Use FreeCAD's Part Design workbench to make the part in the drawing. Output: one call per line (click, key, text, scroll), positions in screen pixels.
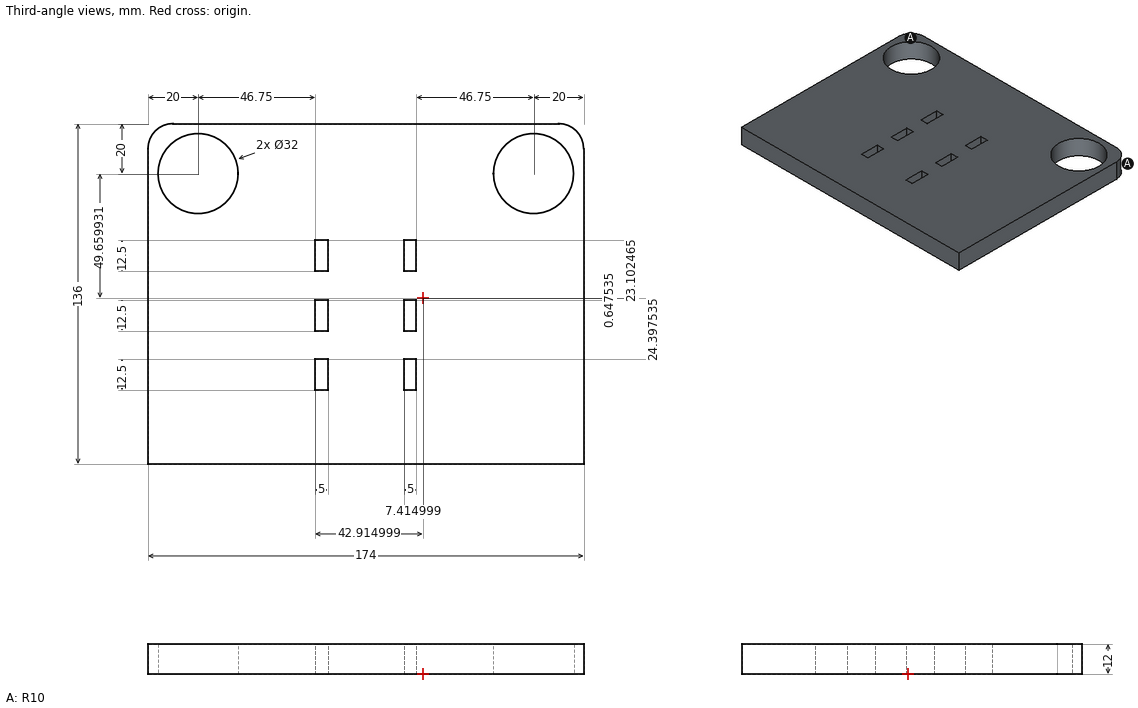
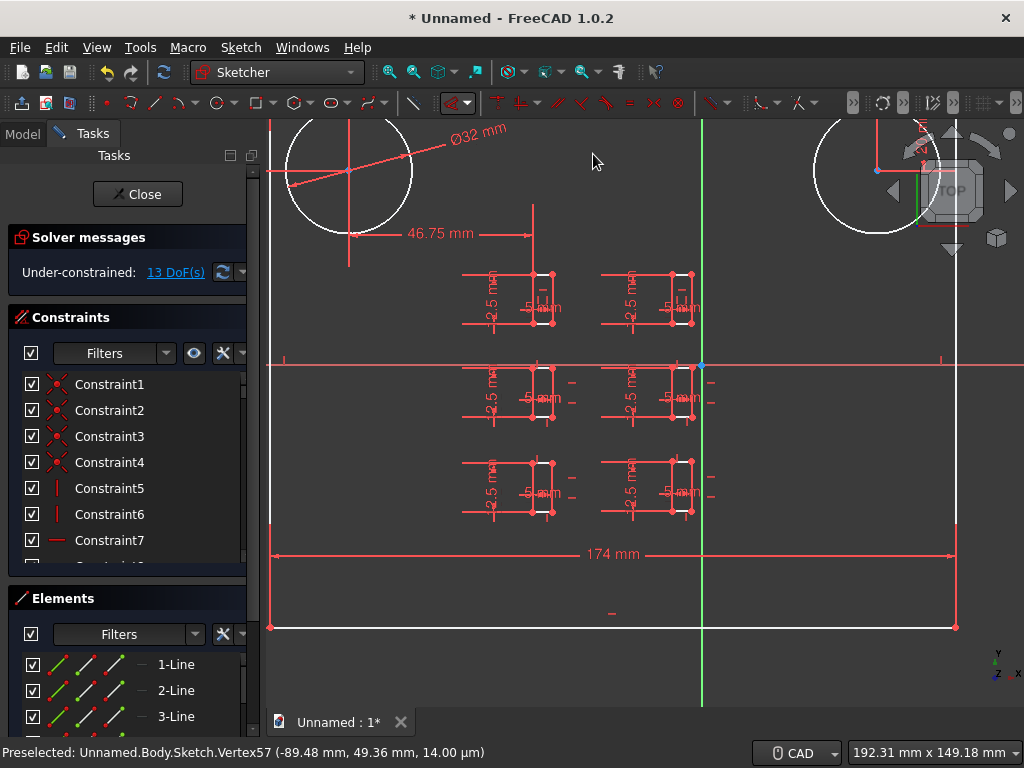
click(692, 275)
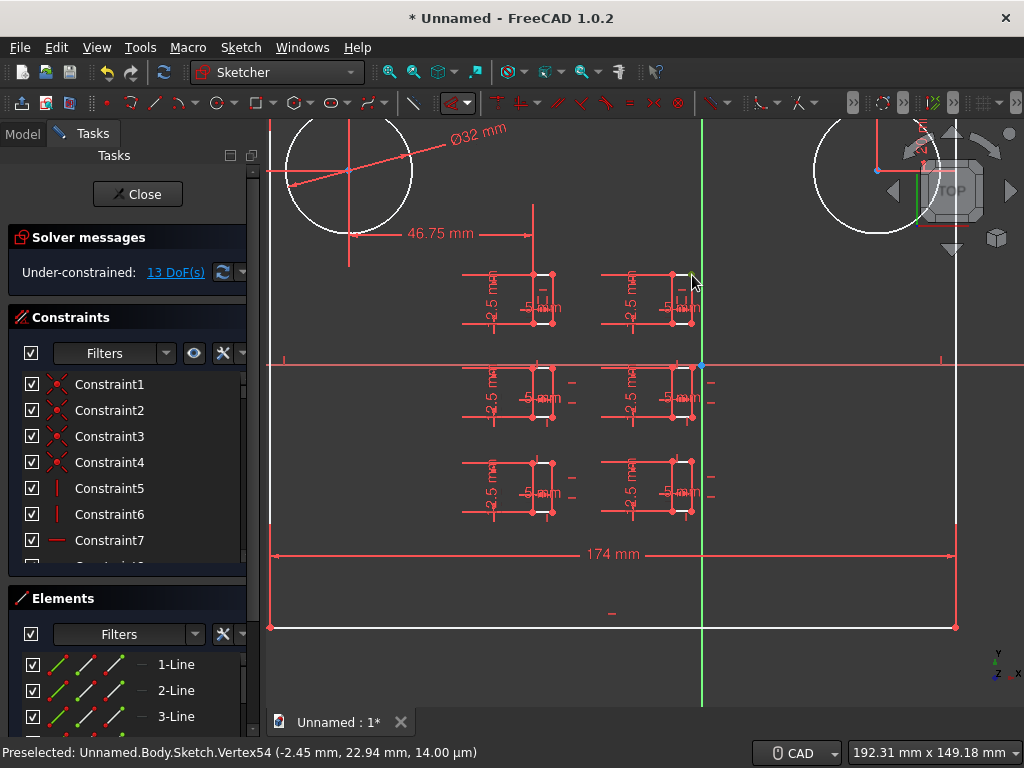
scroll(533, 479, down, 3)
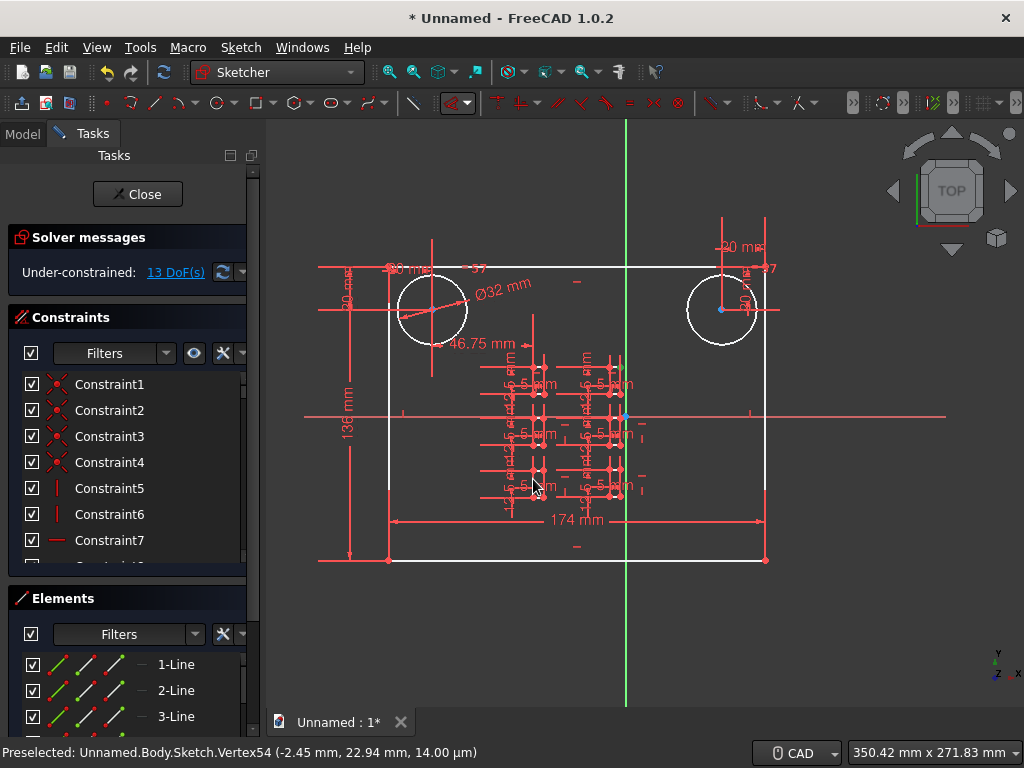
click(722, 310)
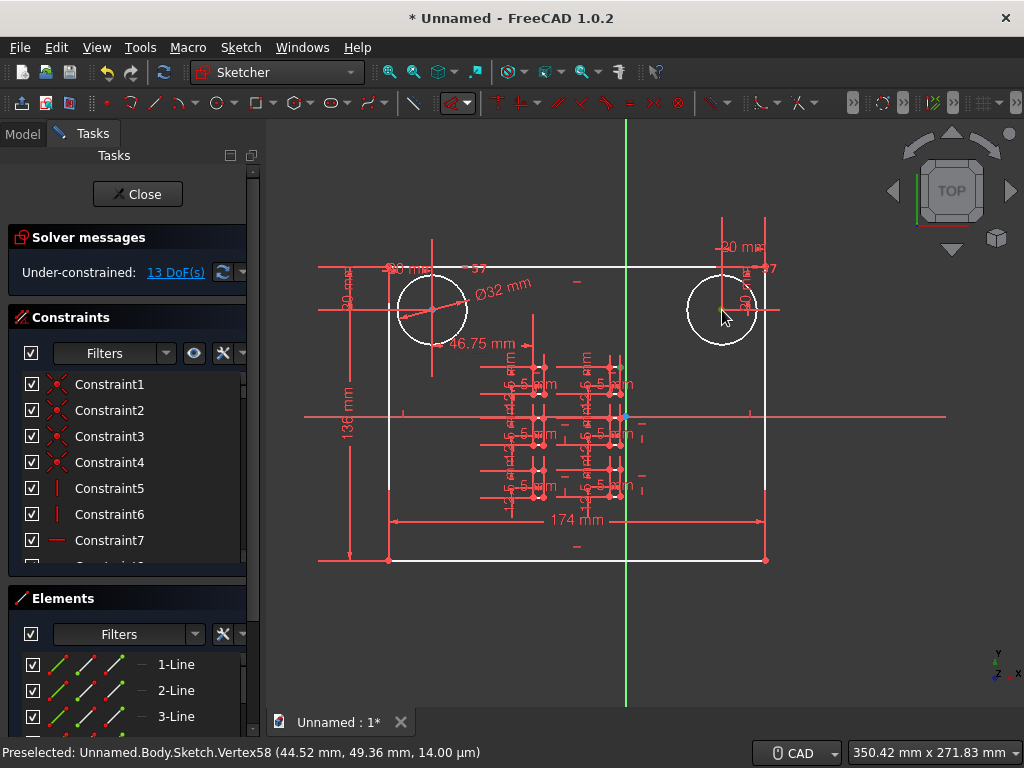
key(l)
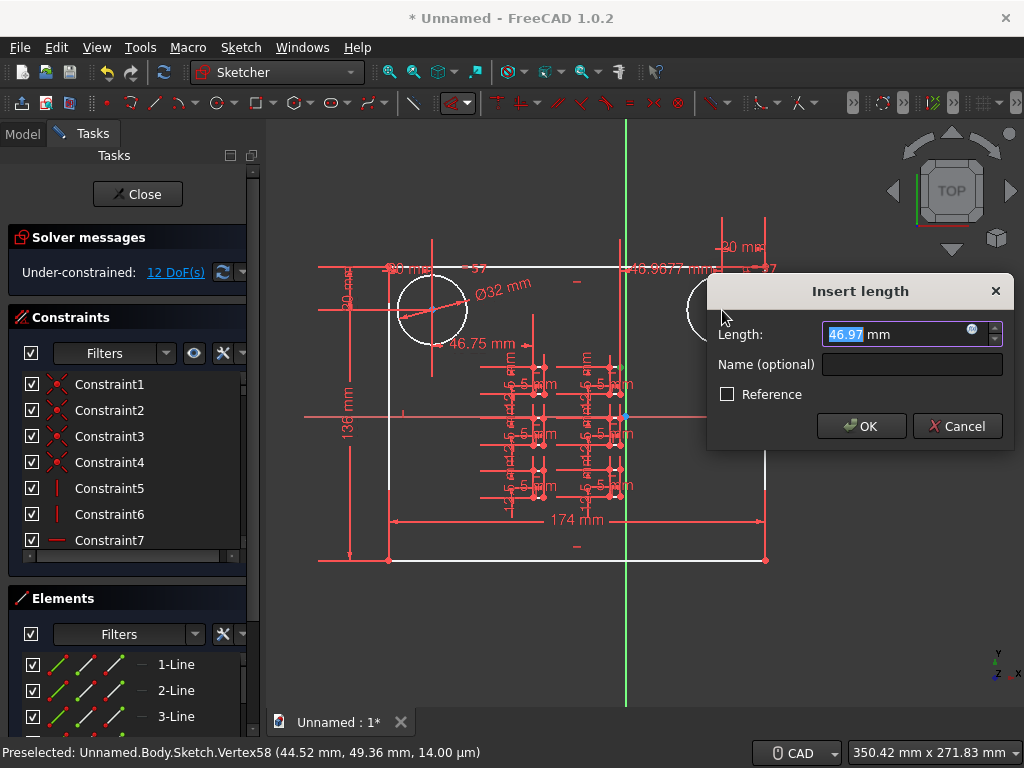
text(46.75)
key(Return)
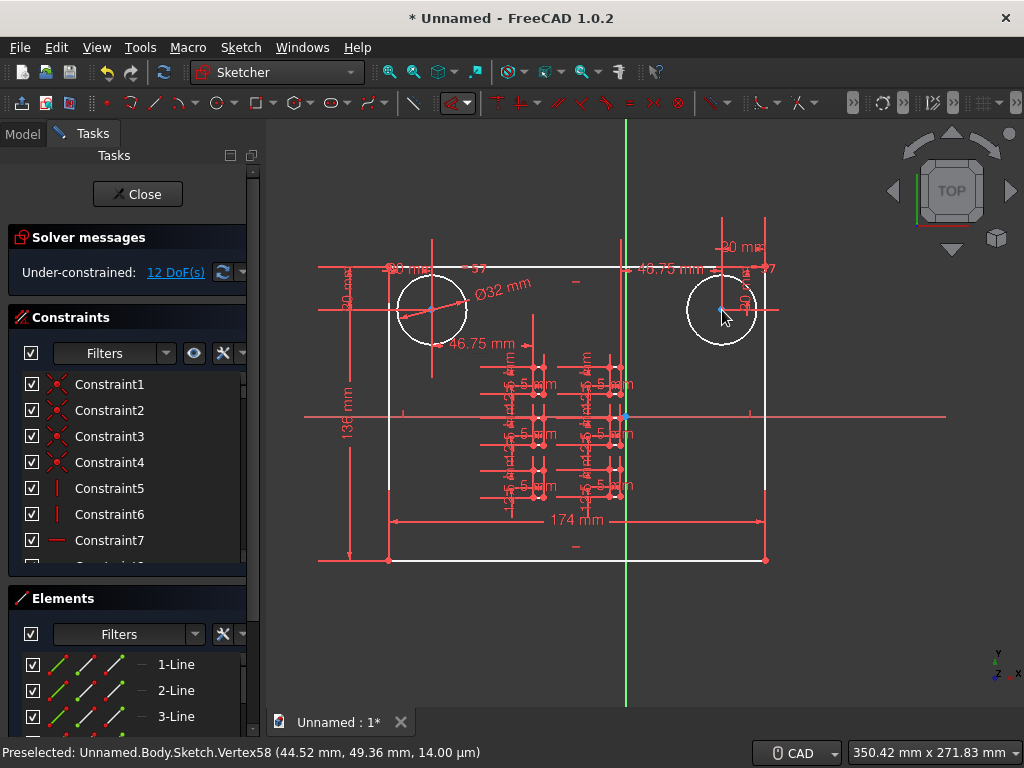
scroll(533, 418, up, 17)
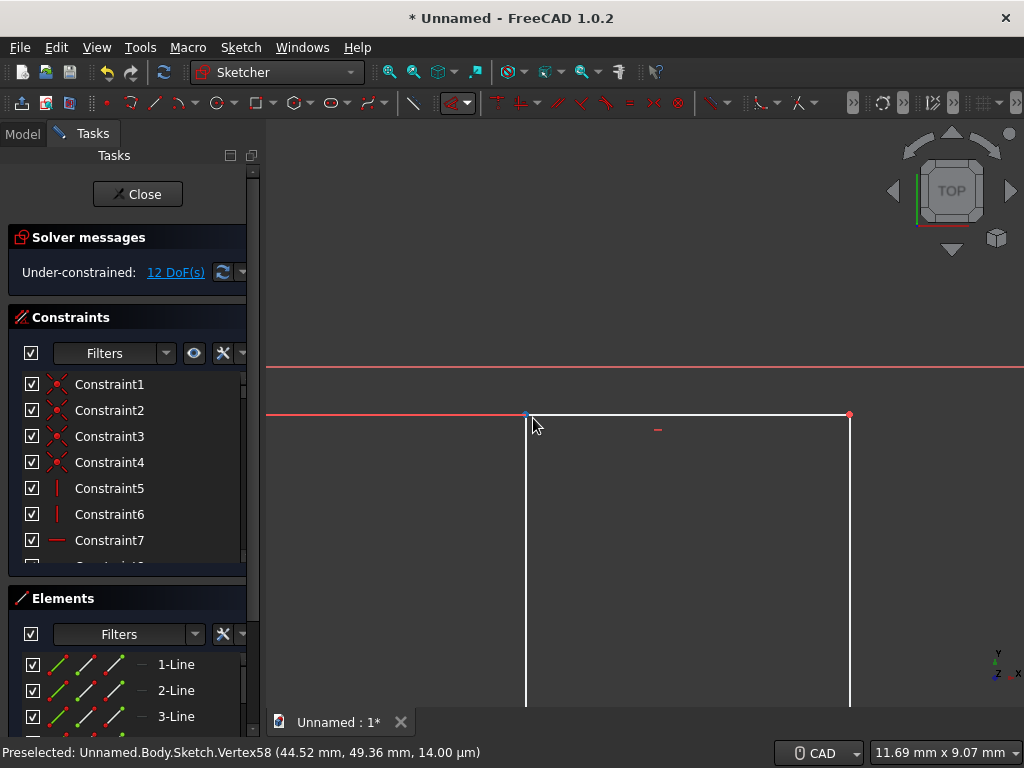
click(526, 415)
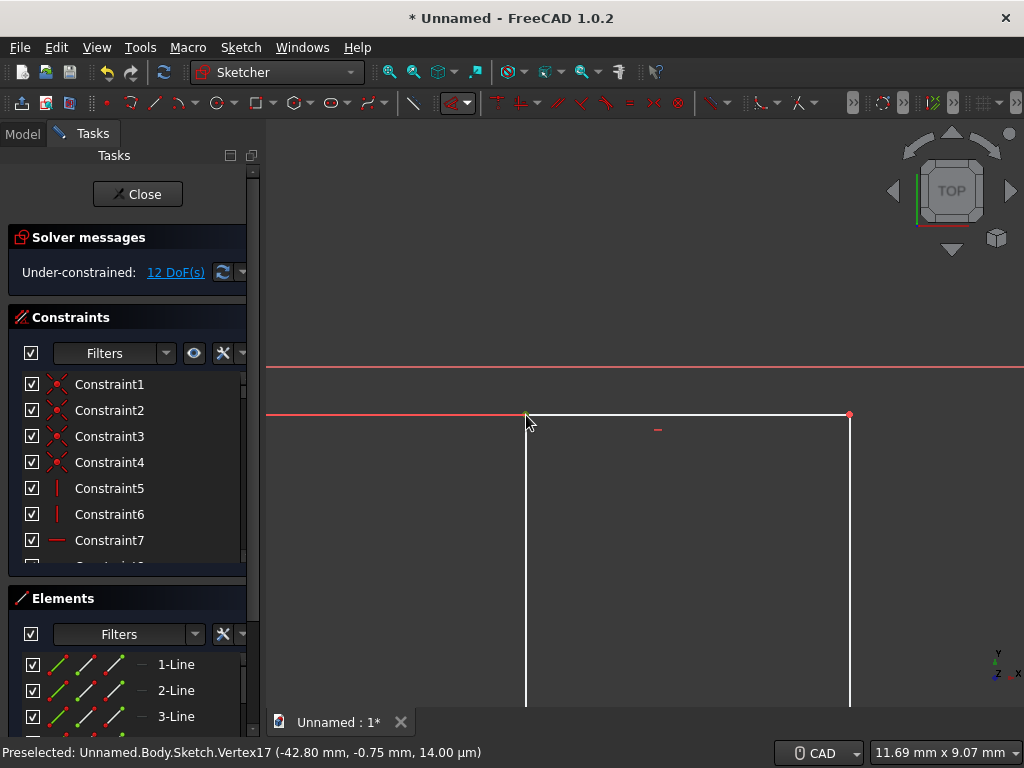
click(470, 104)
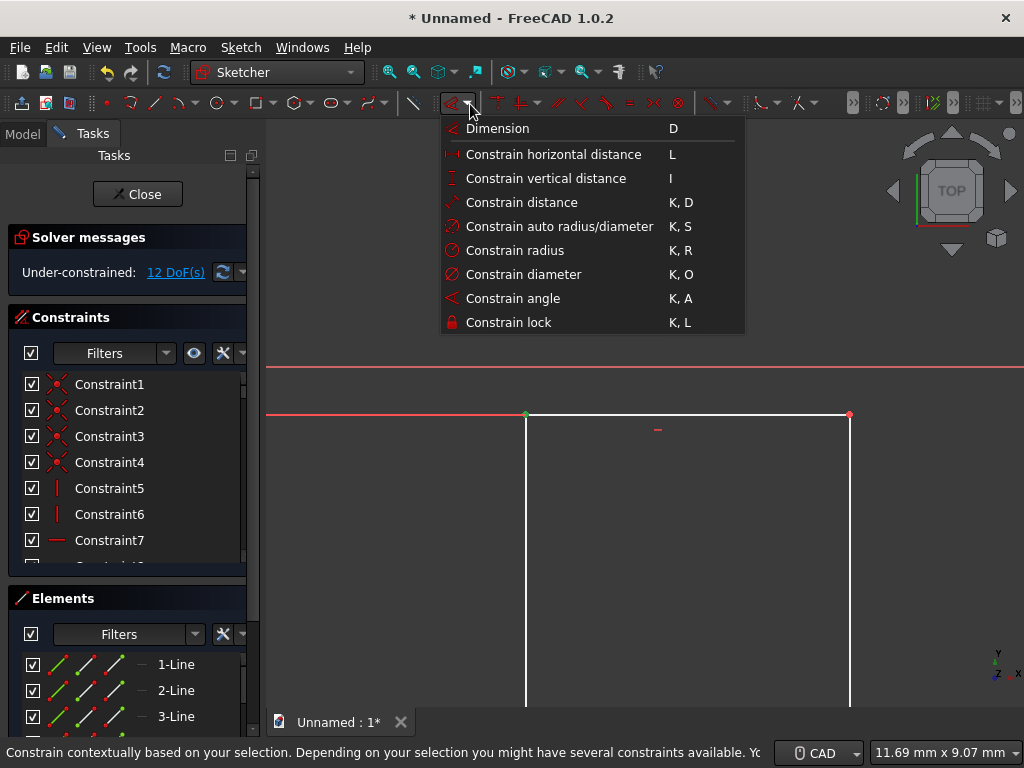
click(593, 178)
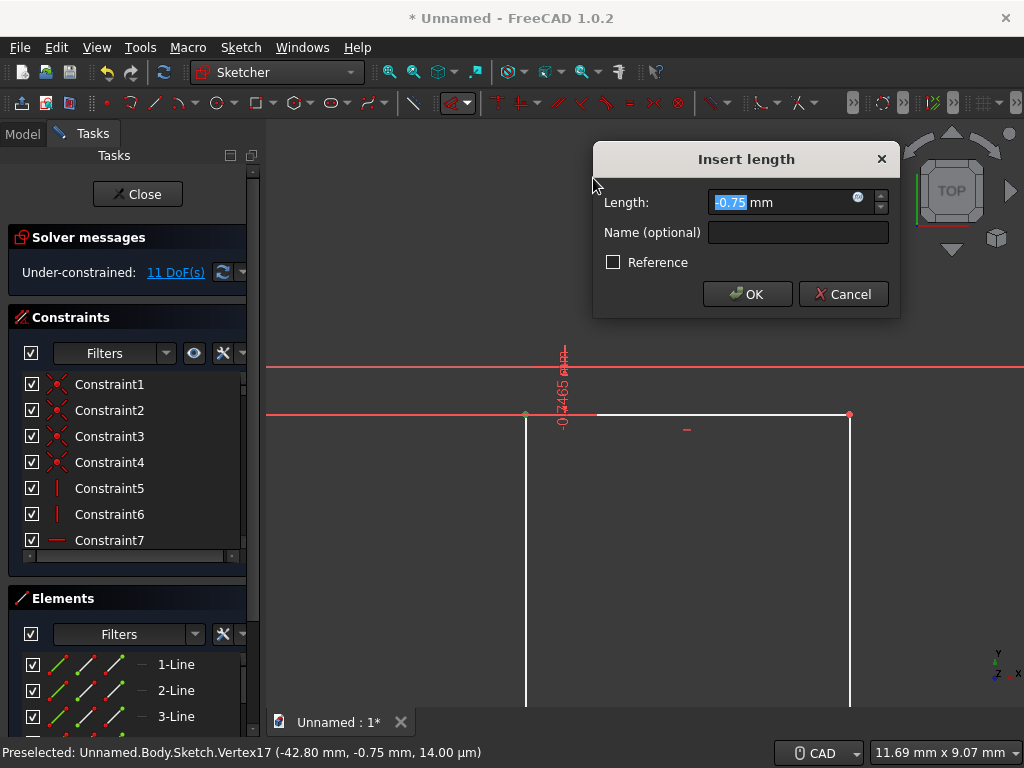
text(-0.647535)
key(Return)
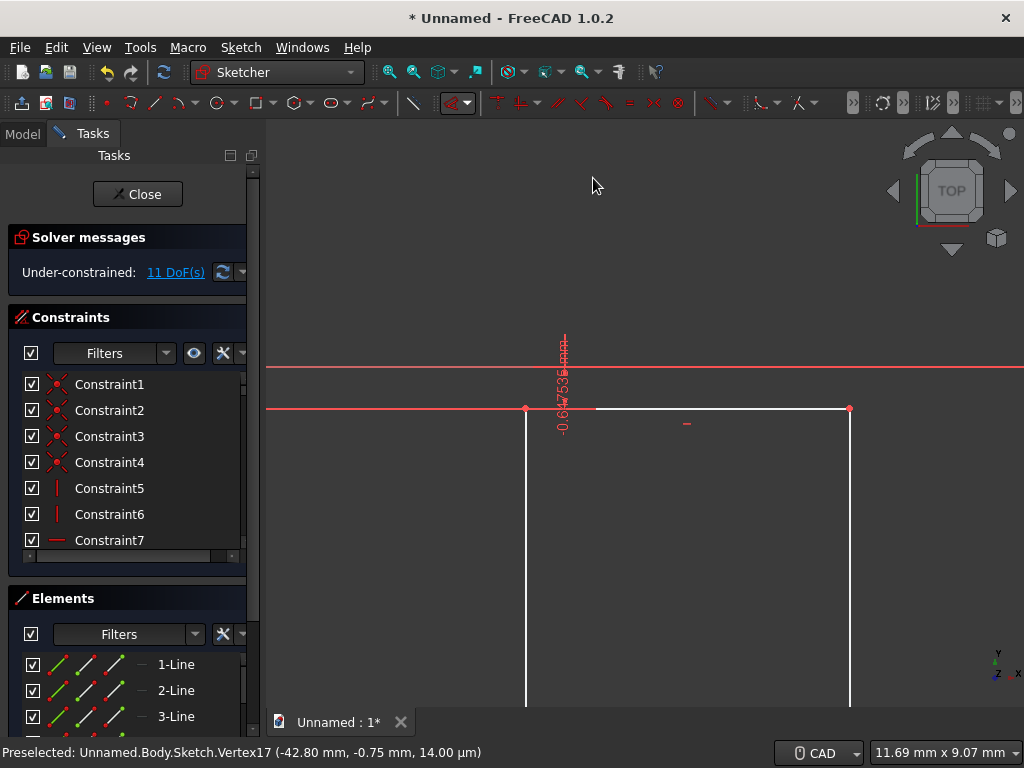
scroll(523, 420, down, 16)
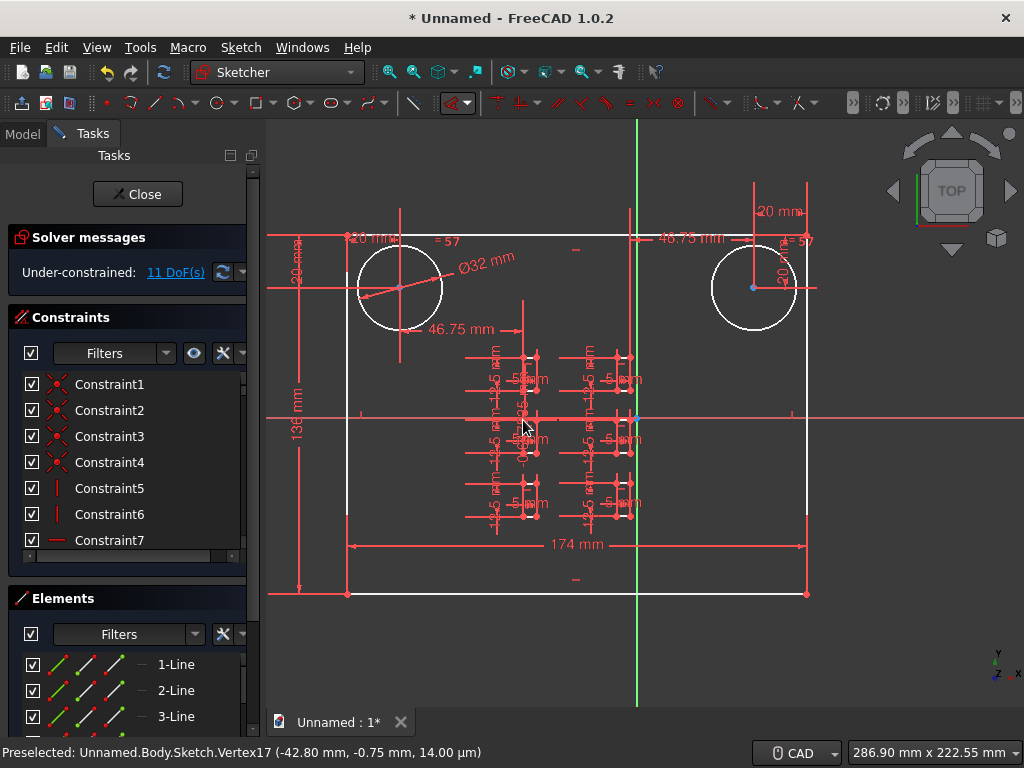
scroll(617, 483, up, 4)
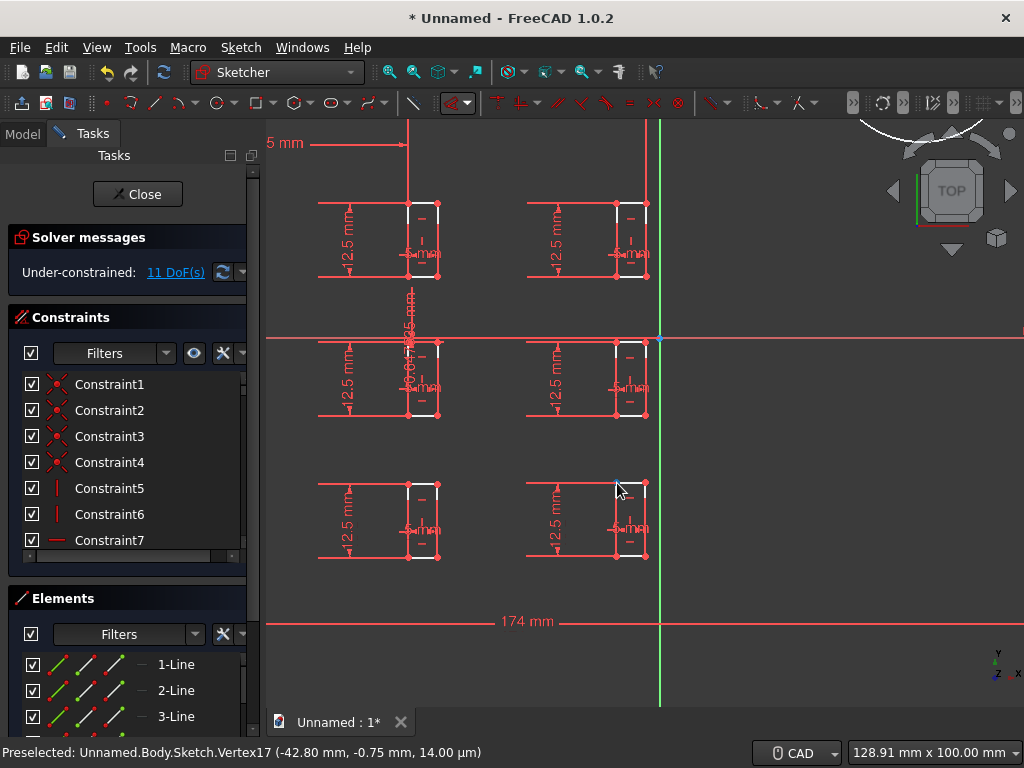
click(616, 483)